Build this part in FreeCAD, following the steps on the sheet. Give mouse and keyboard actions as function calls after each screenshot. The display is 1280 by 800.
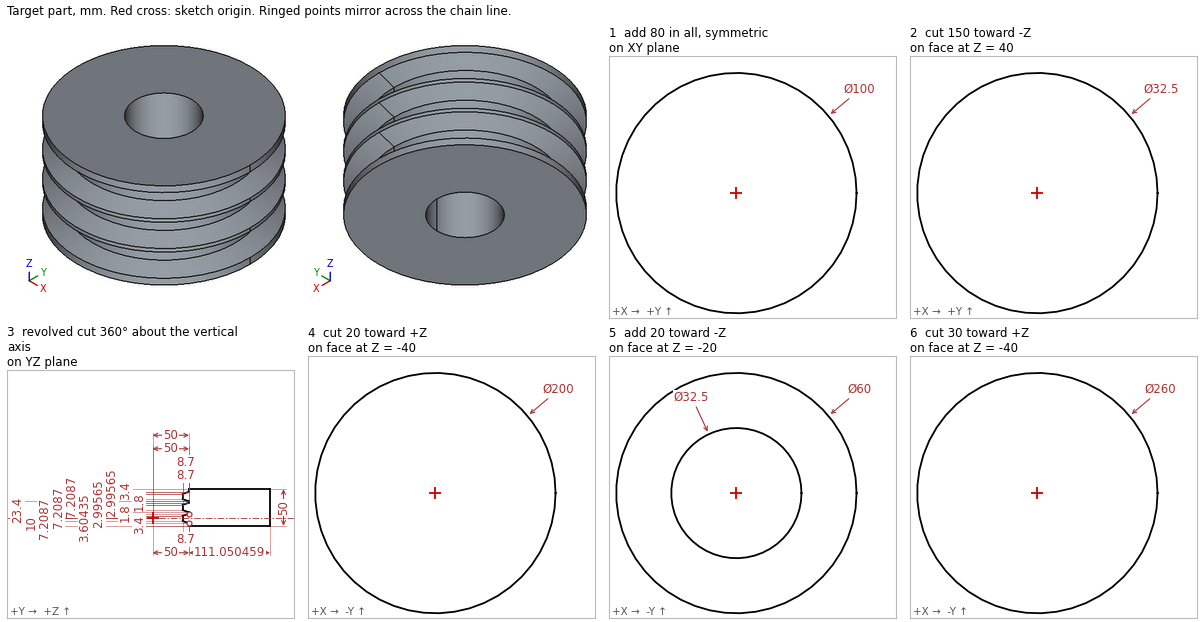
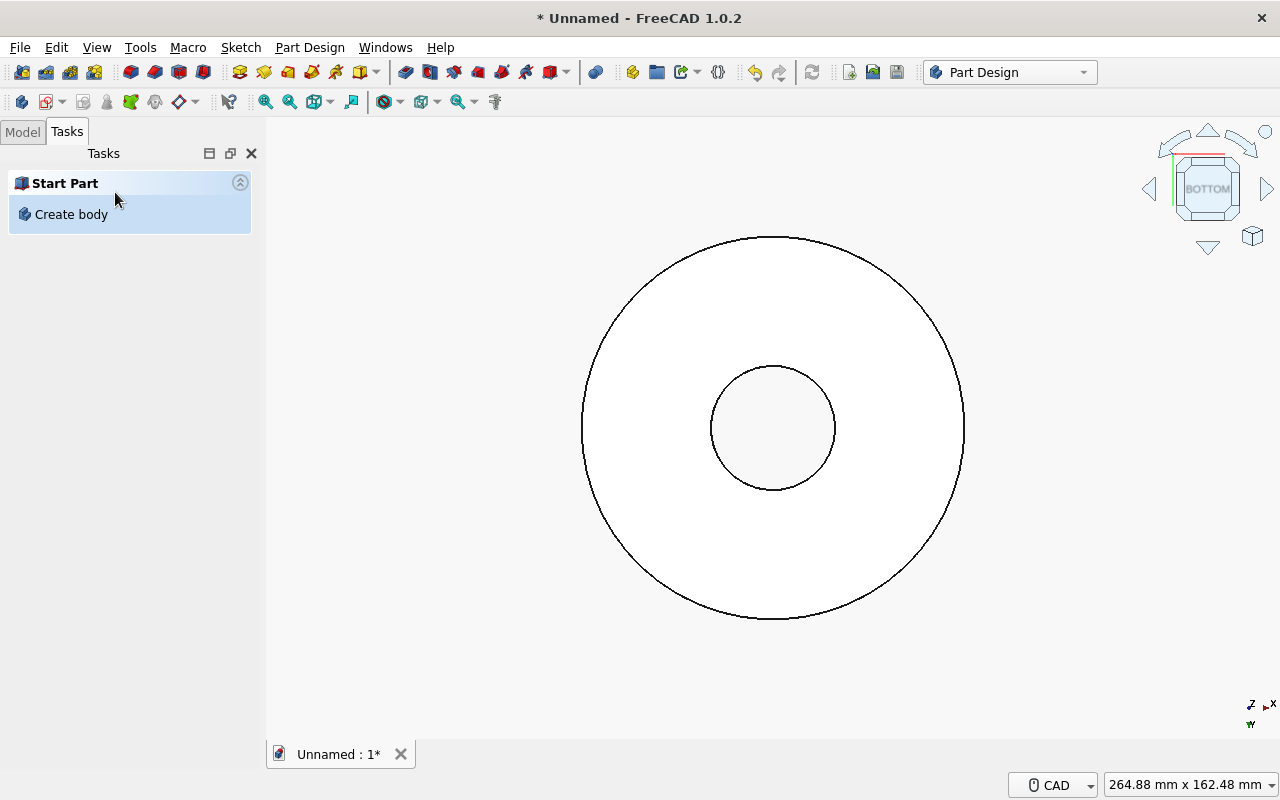
click(664, 482)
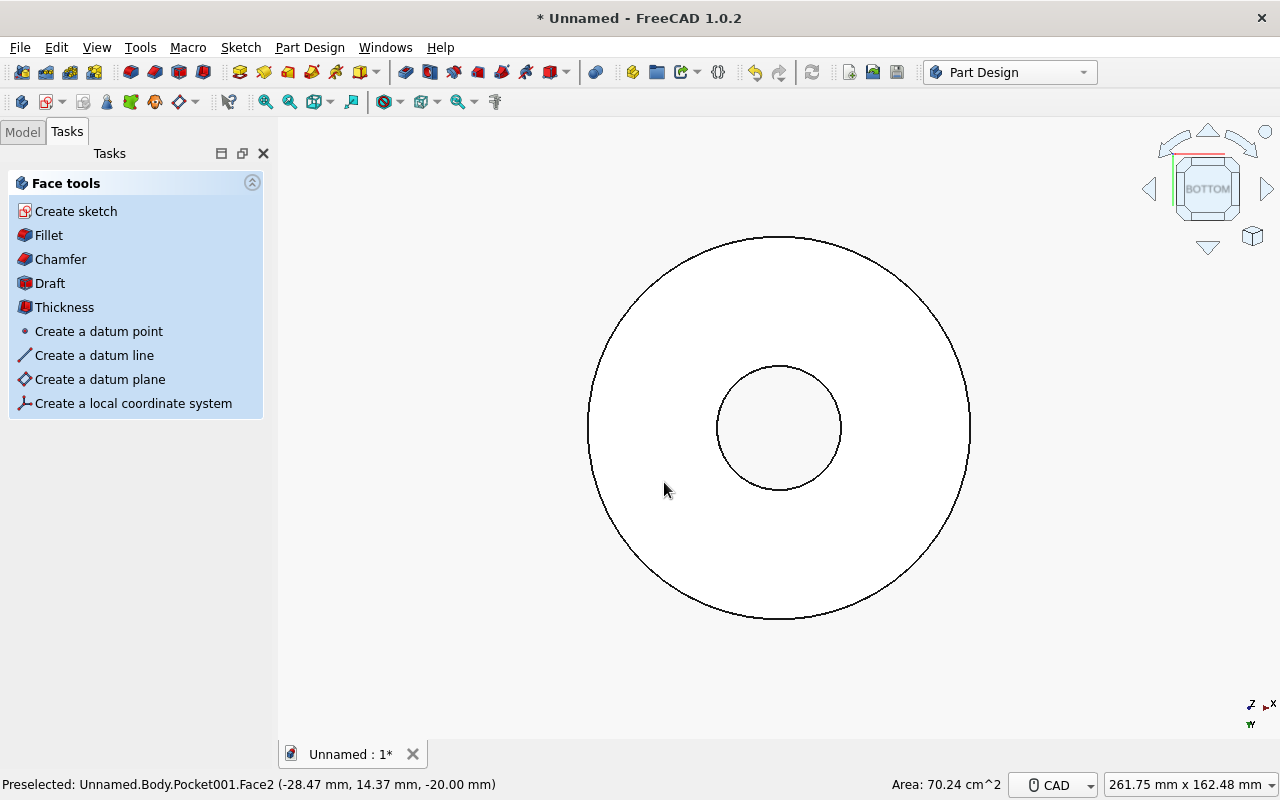
click(46, 102)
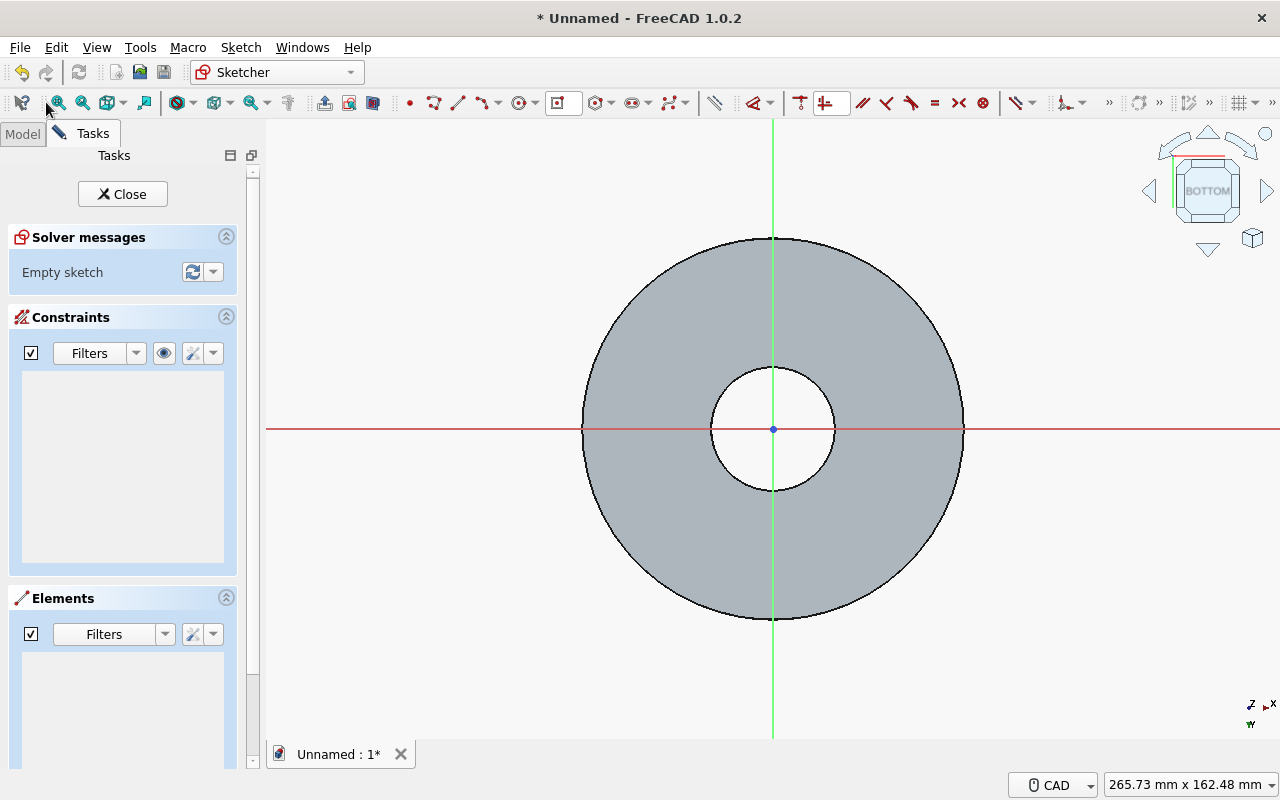
scroll(856, 429, up, 3)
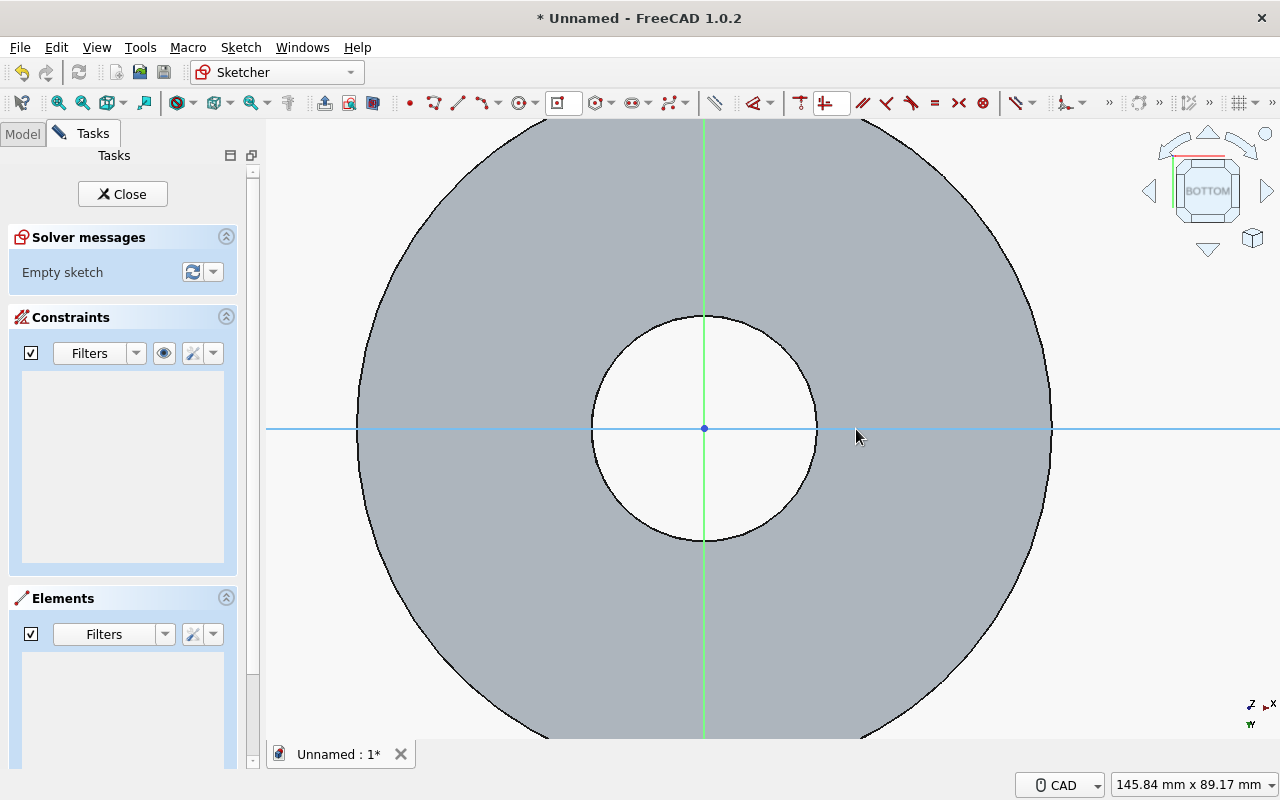
click(520, 104)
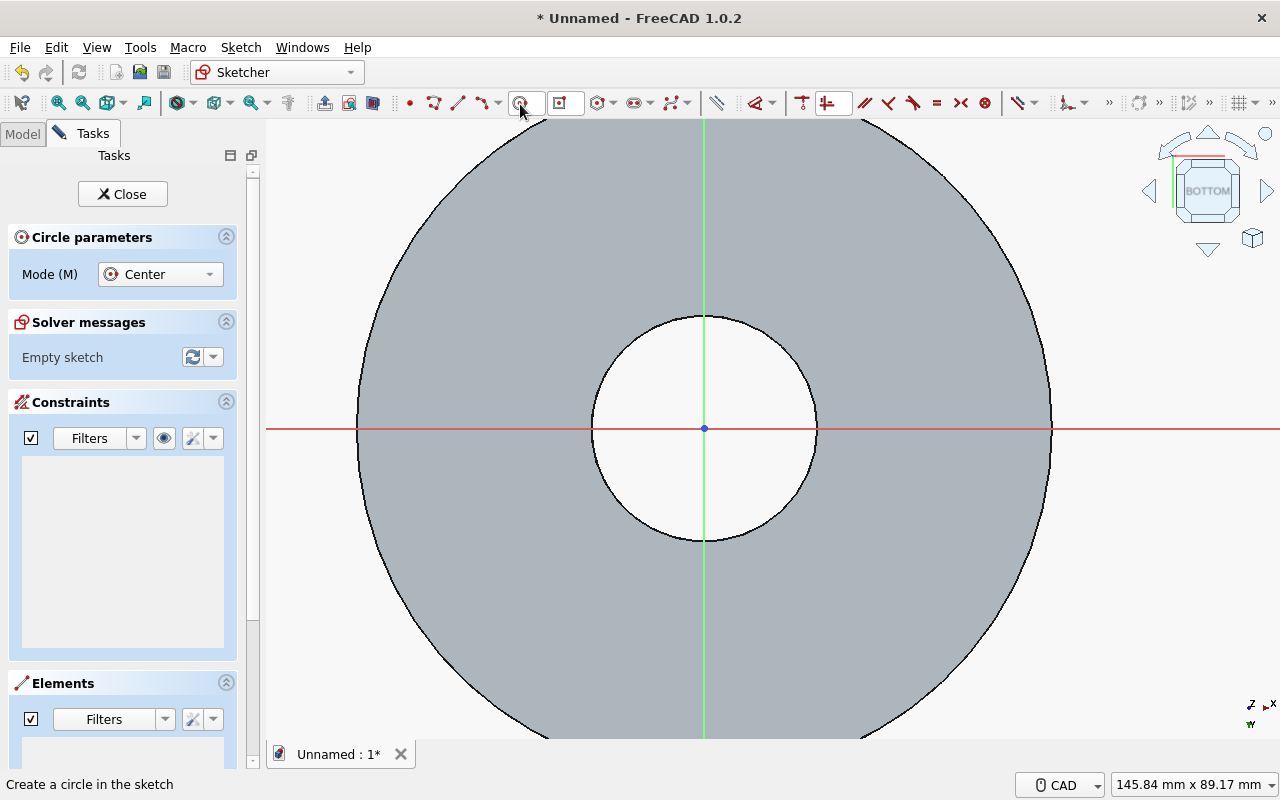
click(704, 429)
click(852, 281)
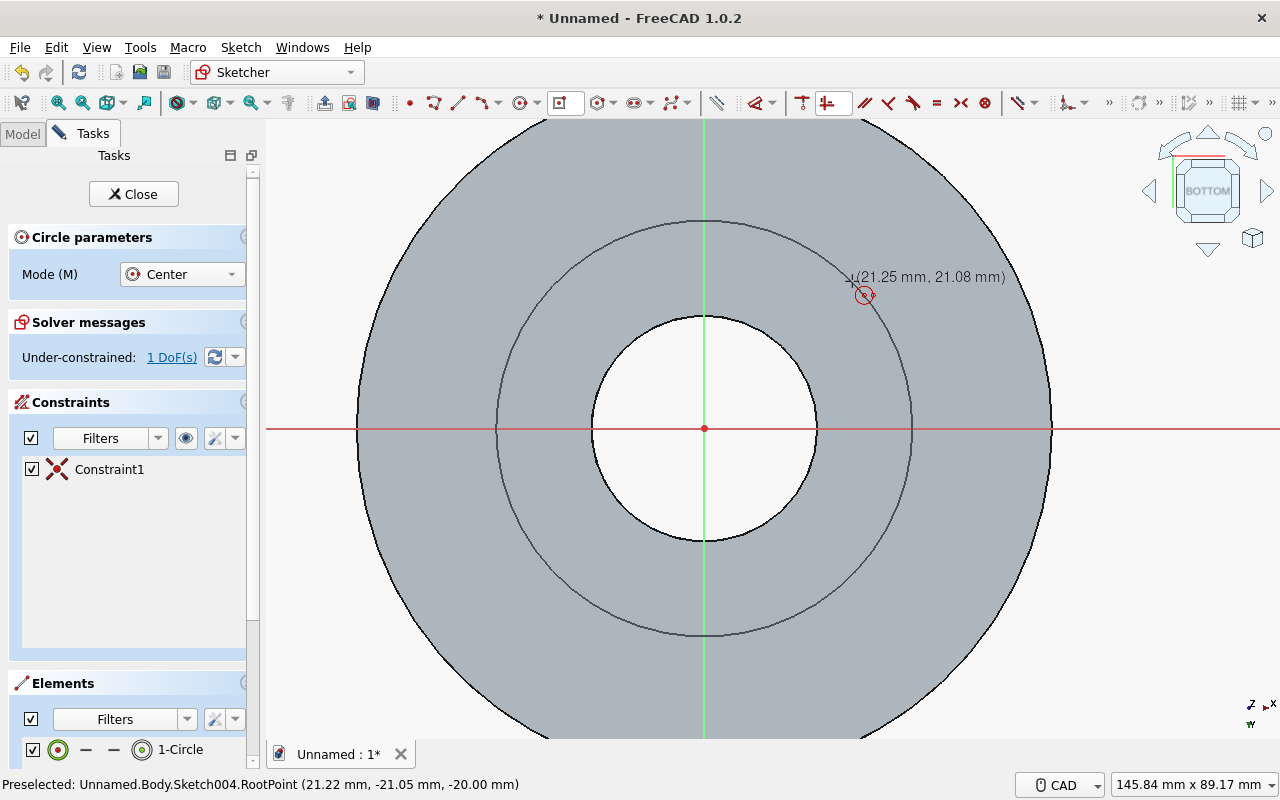
click(704, 429)
click(784, 349)
key(Escape)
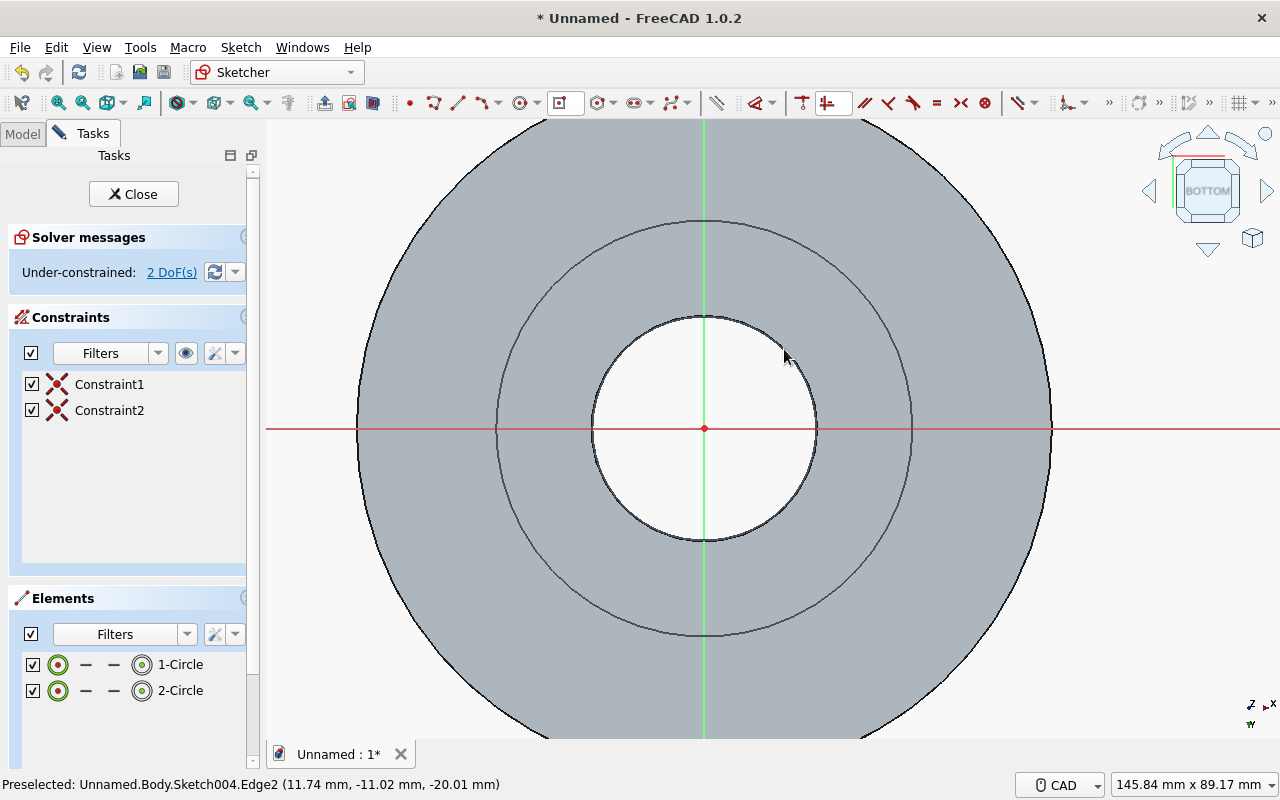
click(756, 104)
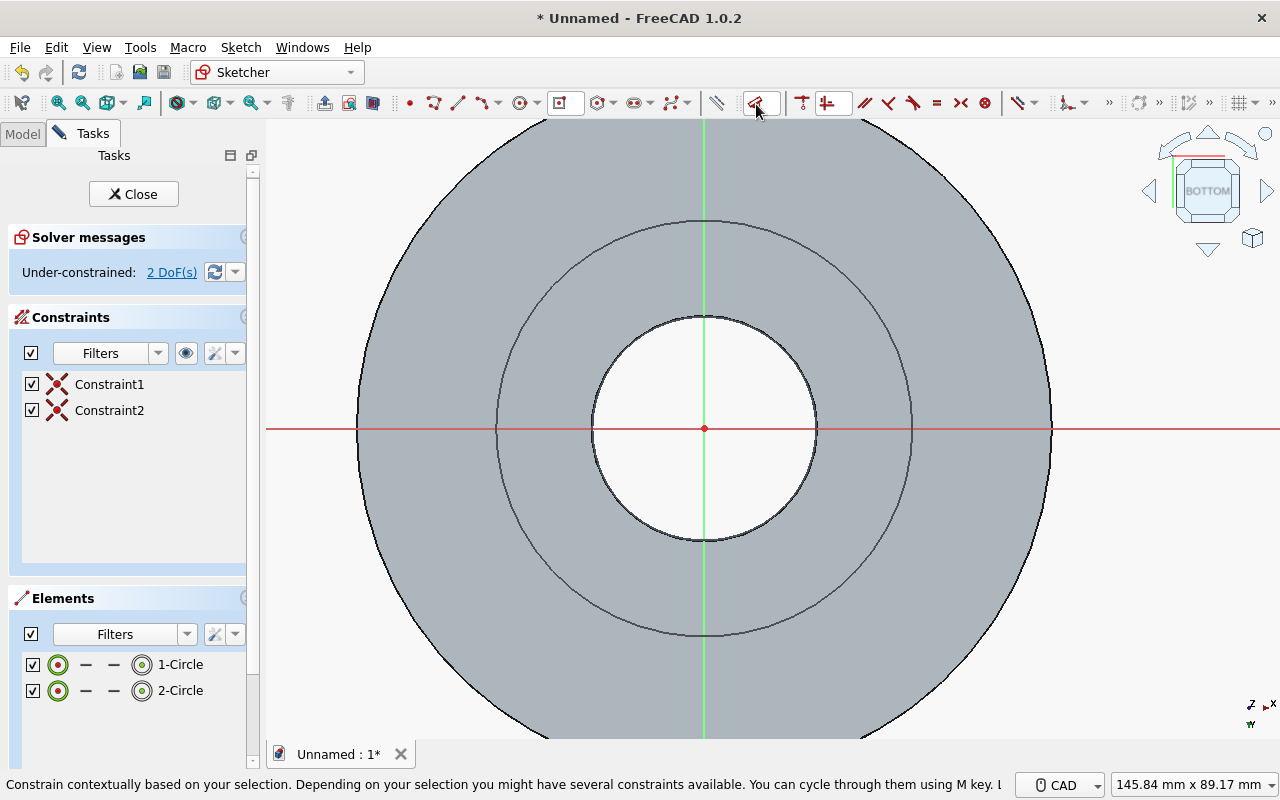
click(851, 281)
click(874, 258)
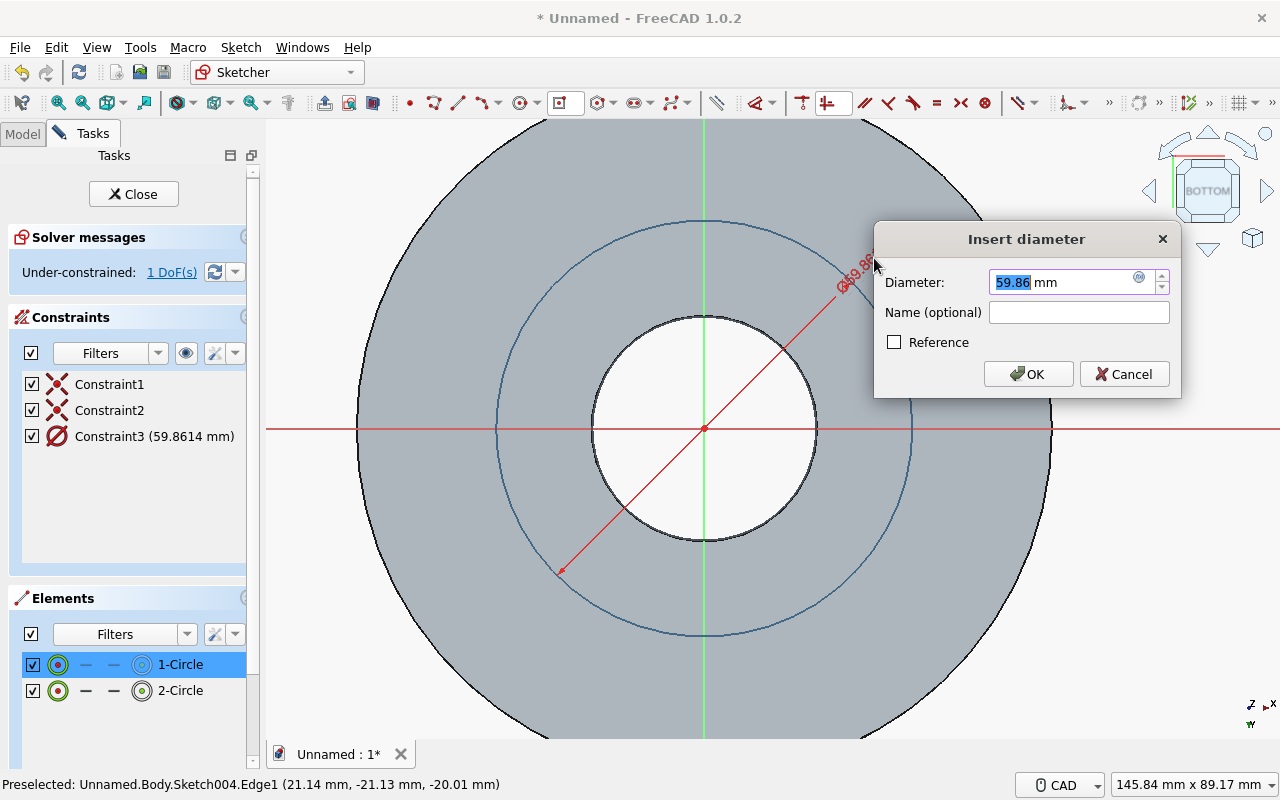
text(60)
key(Return)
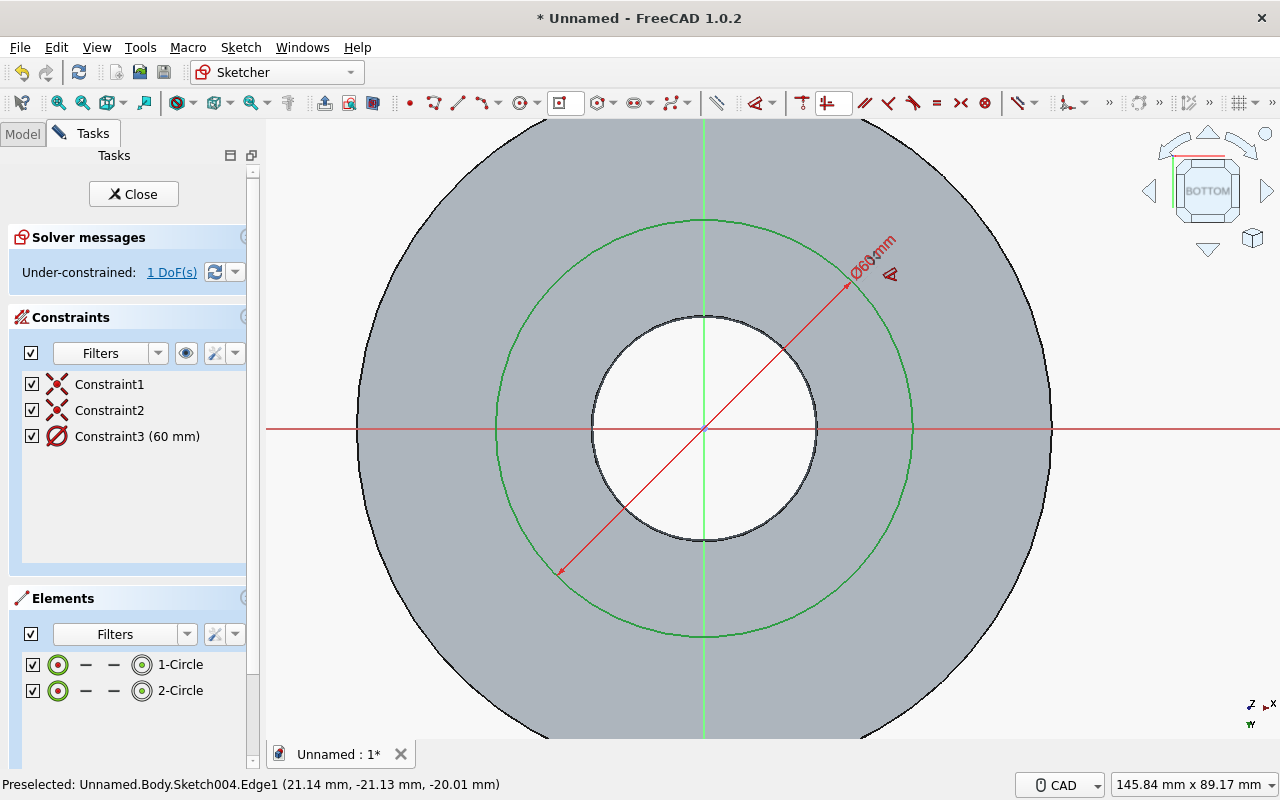
click(783, 349)
click(806, 326)